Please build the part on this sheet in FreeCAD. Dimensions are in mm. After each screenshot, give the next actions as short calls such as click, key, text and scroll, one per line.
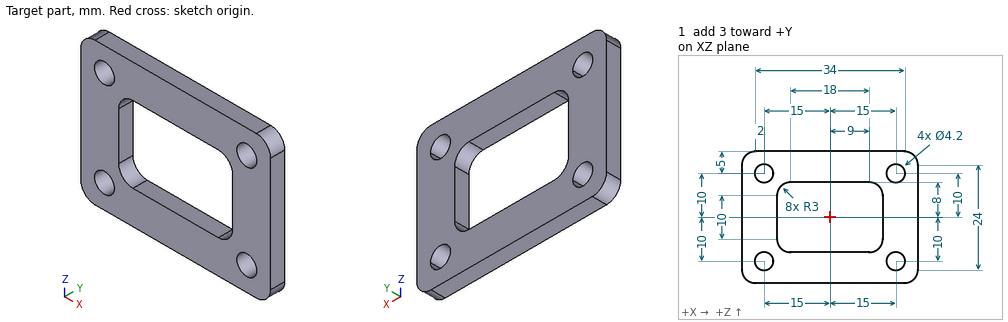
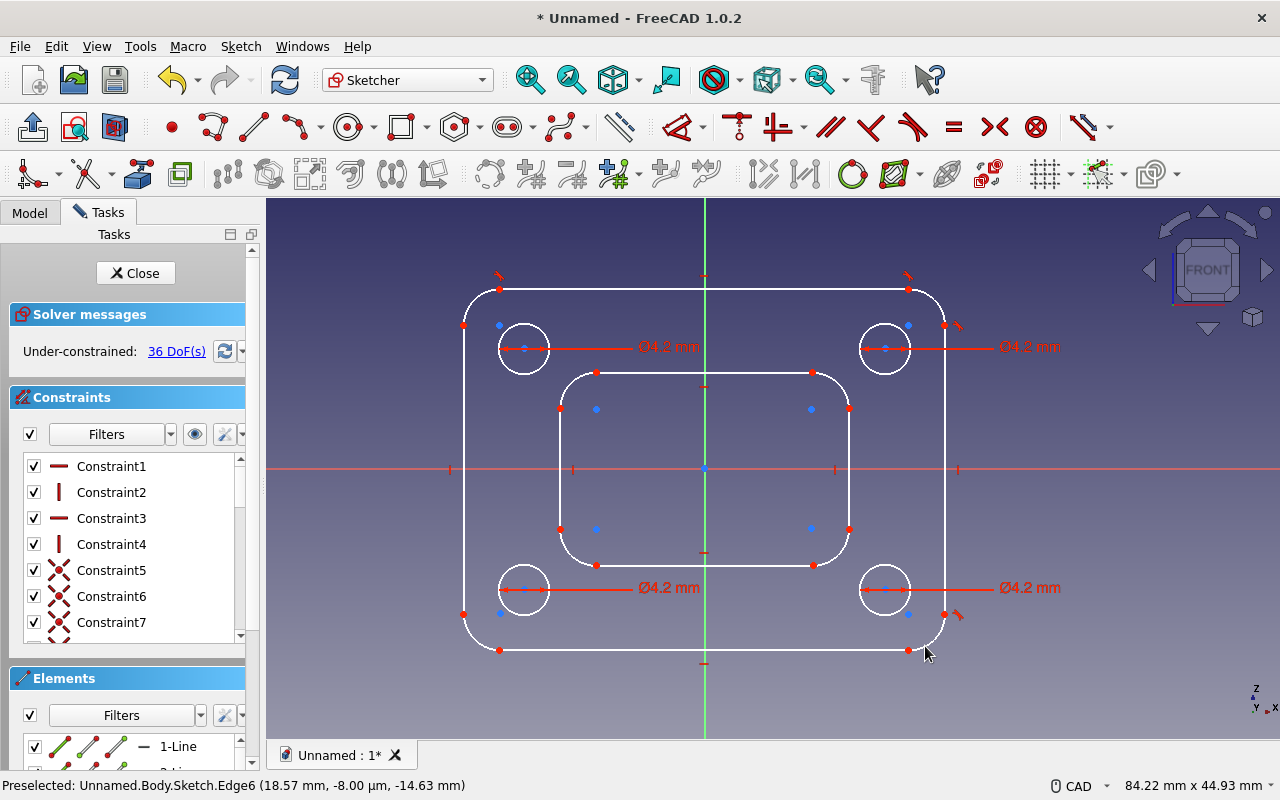
click(786, 650)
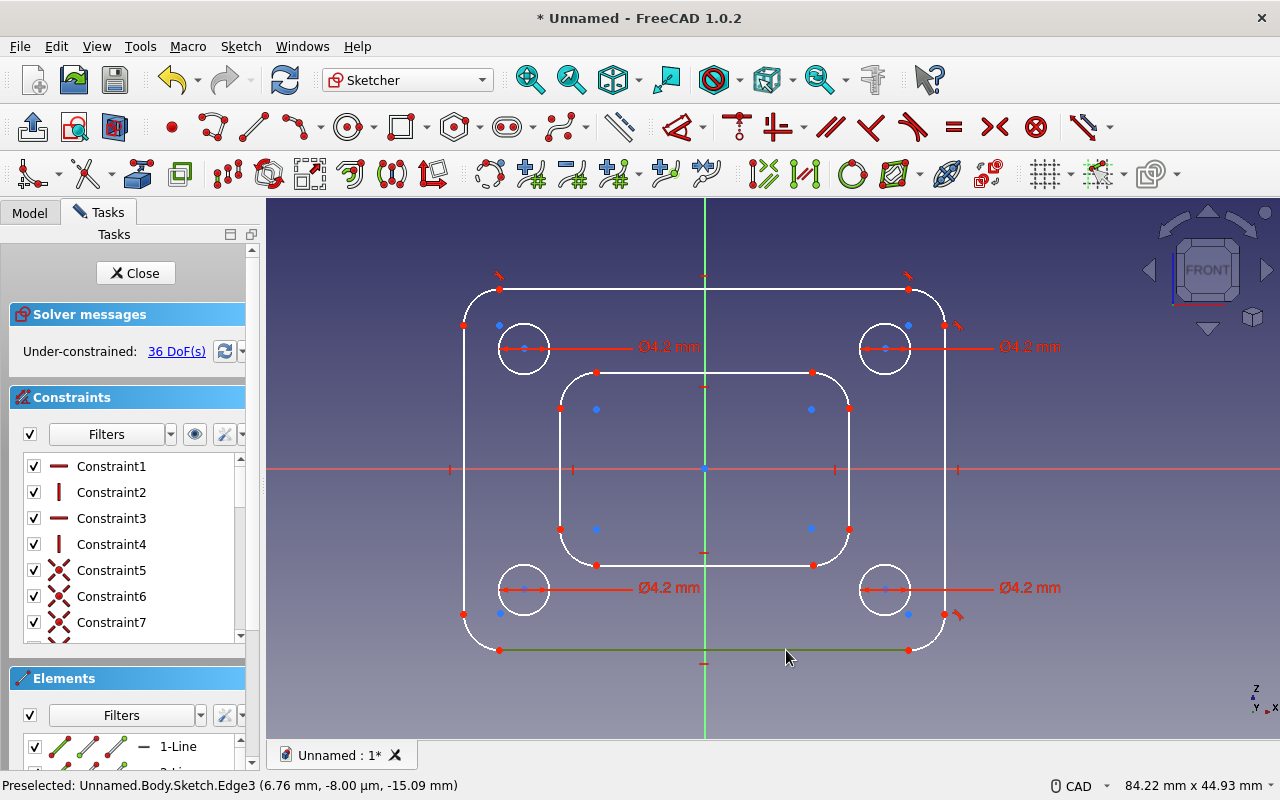
click(925, 646)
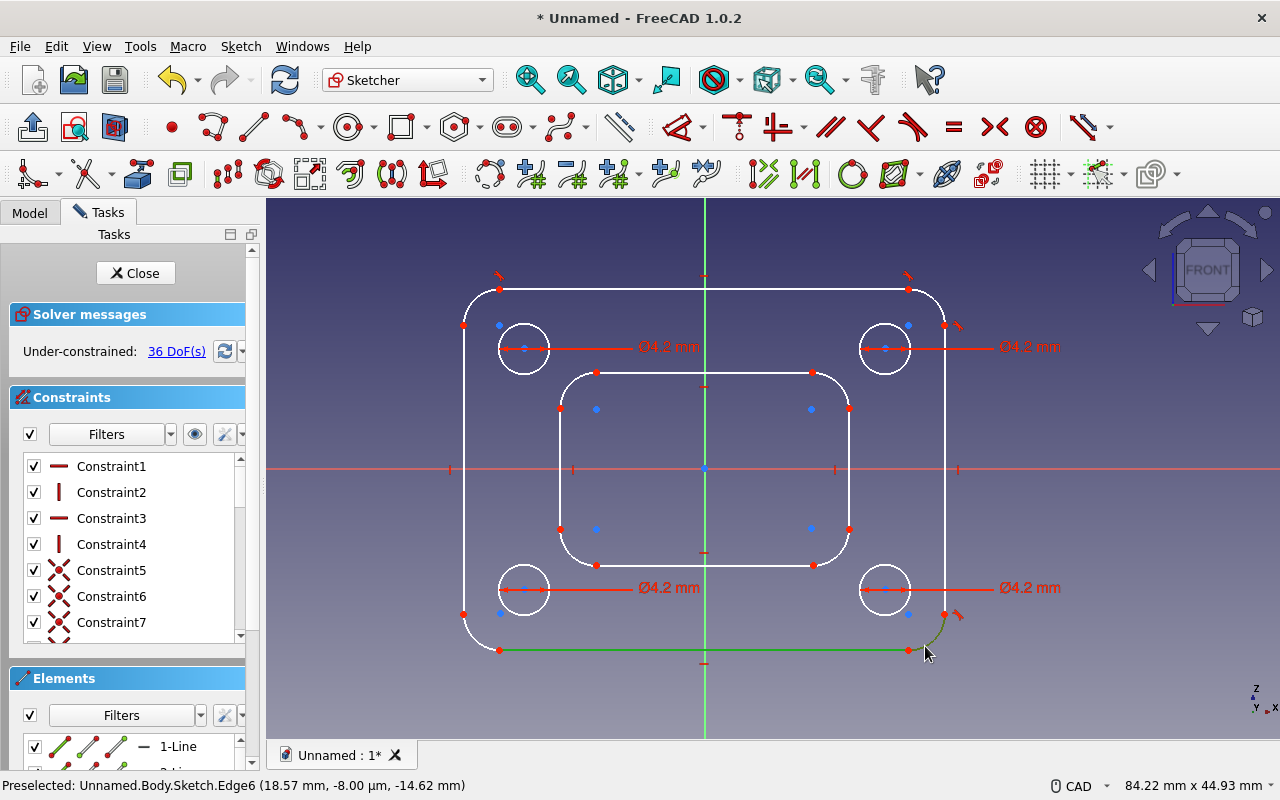
click(913, 128)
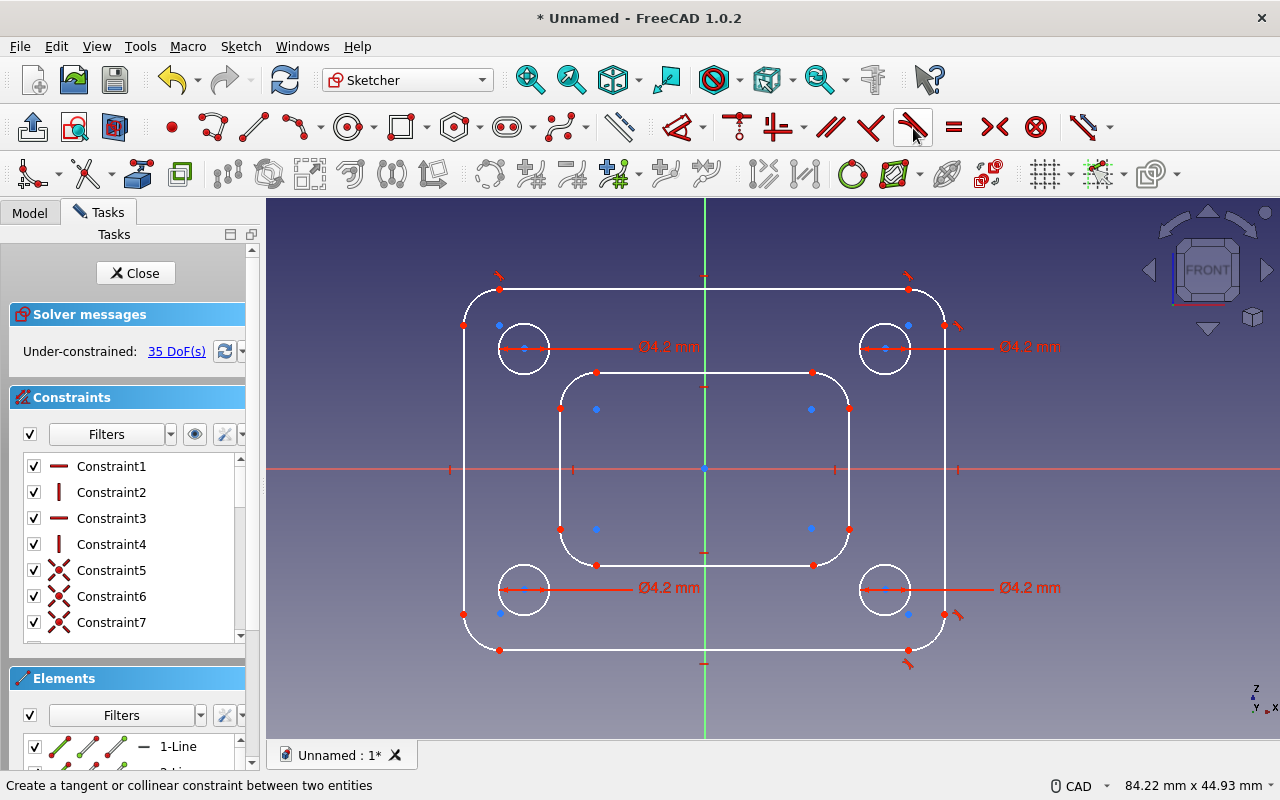
click(786, 650)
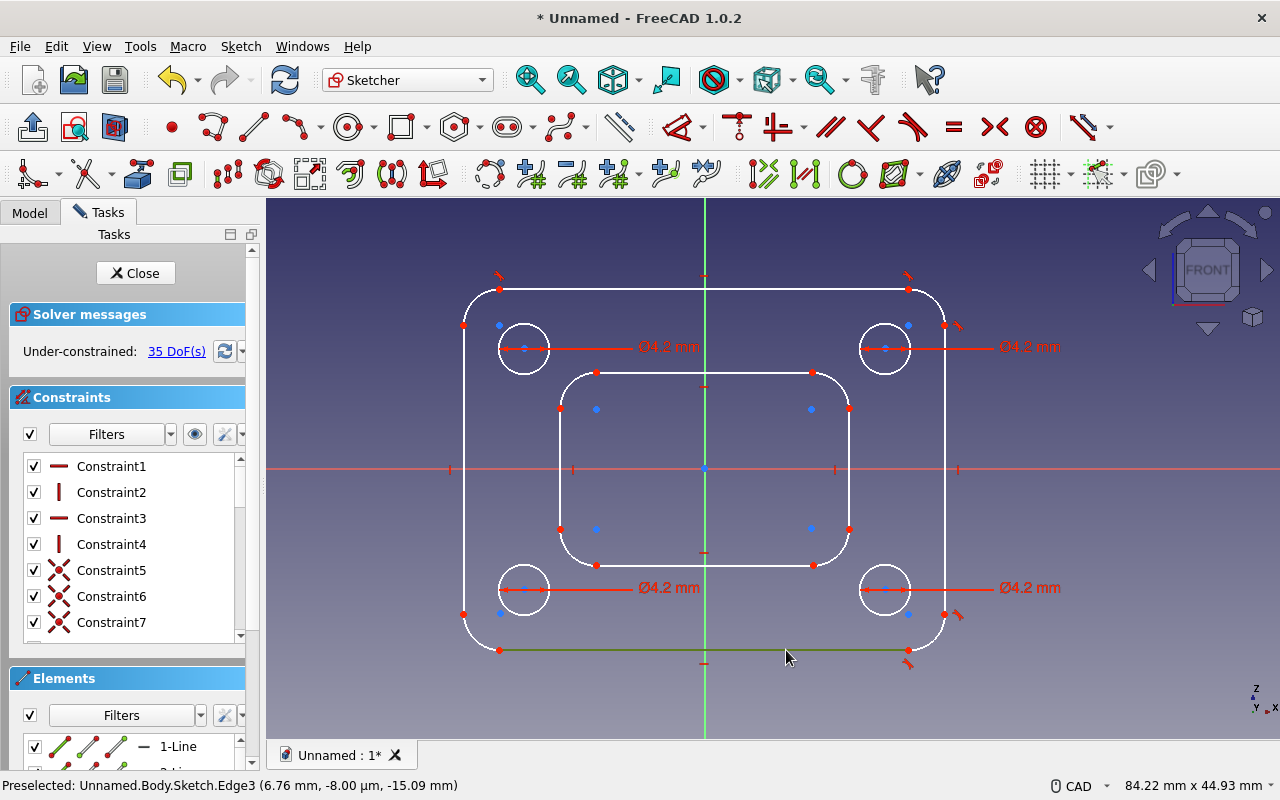
click(468, 631)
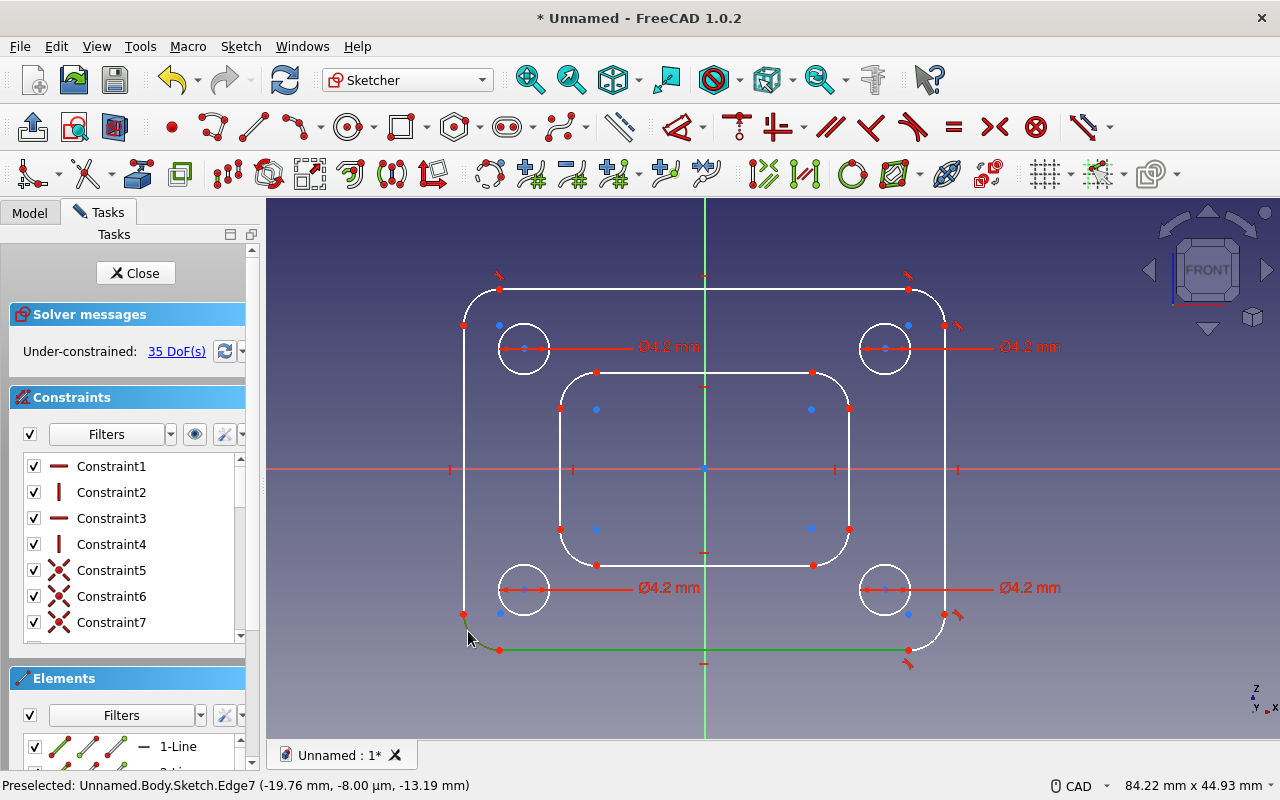
key(t)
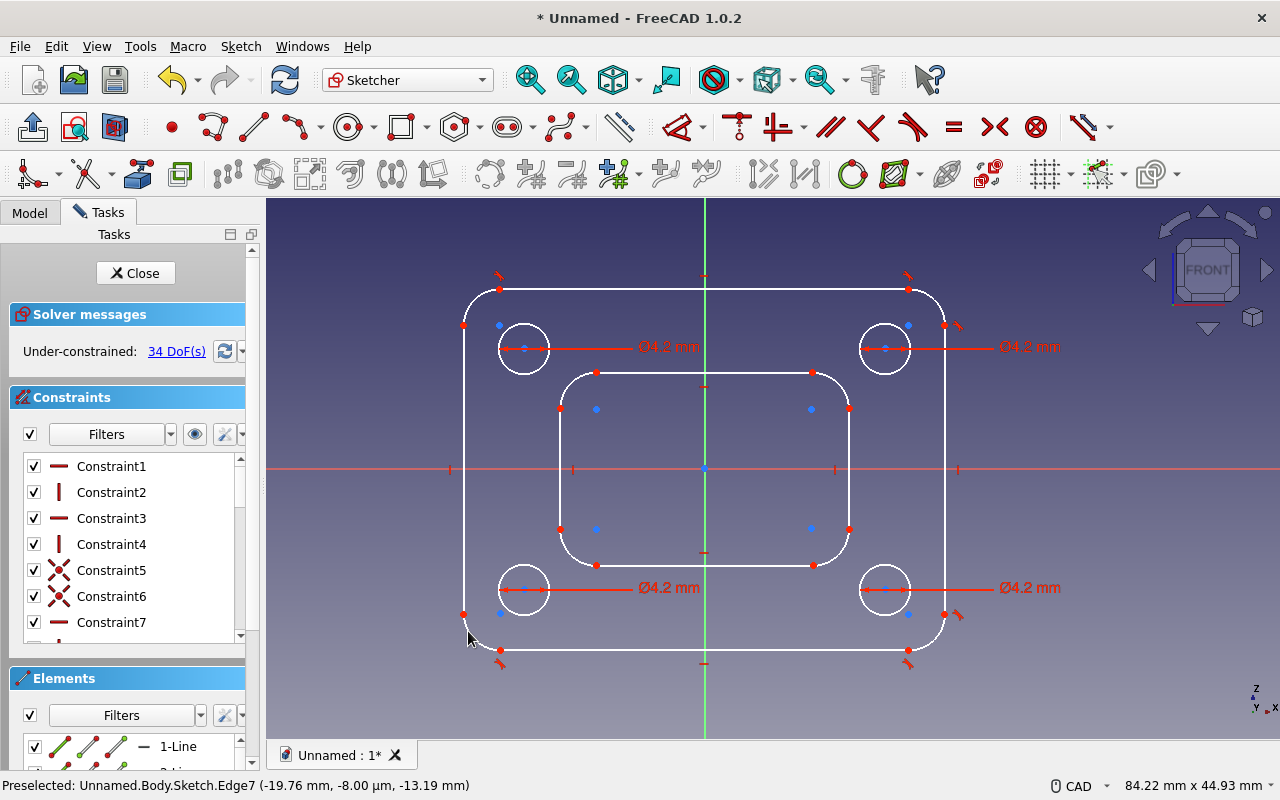
click(464, 528)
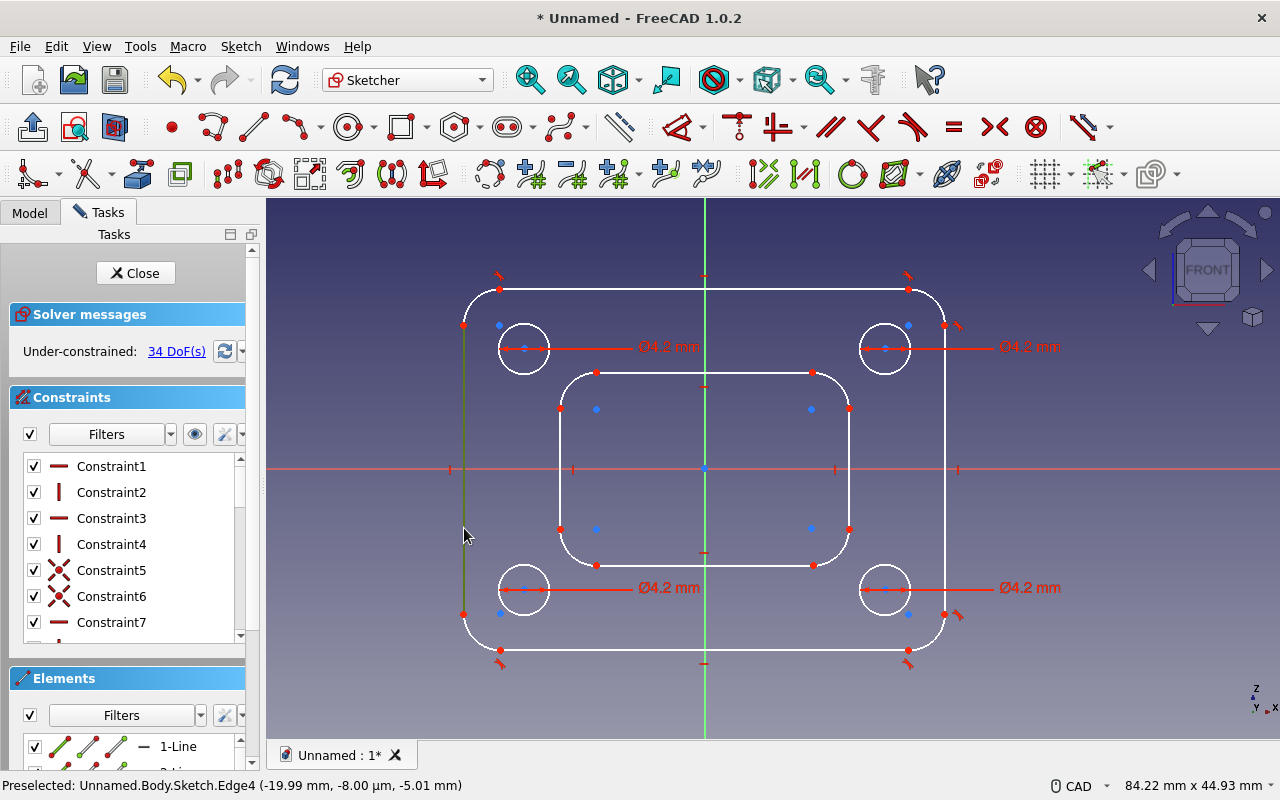
click(468, 631)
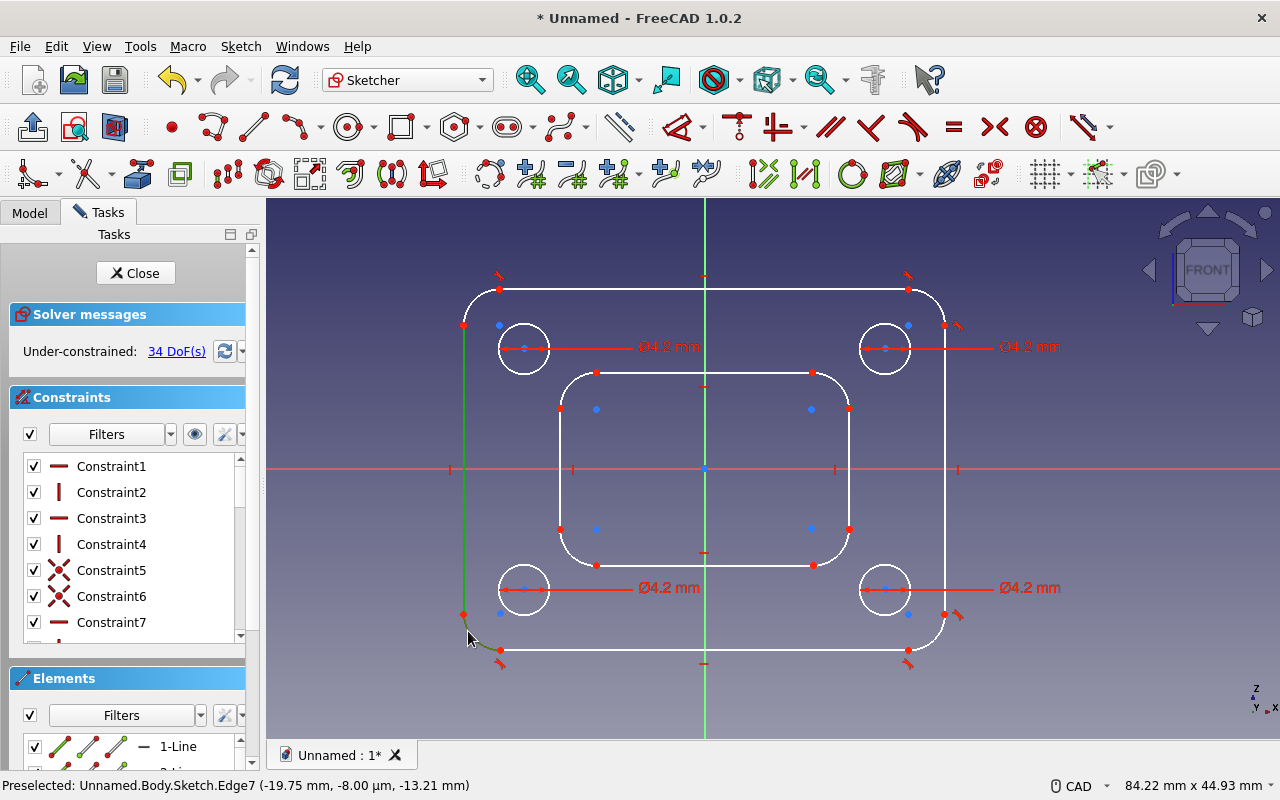
key(t)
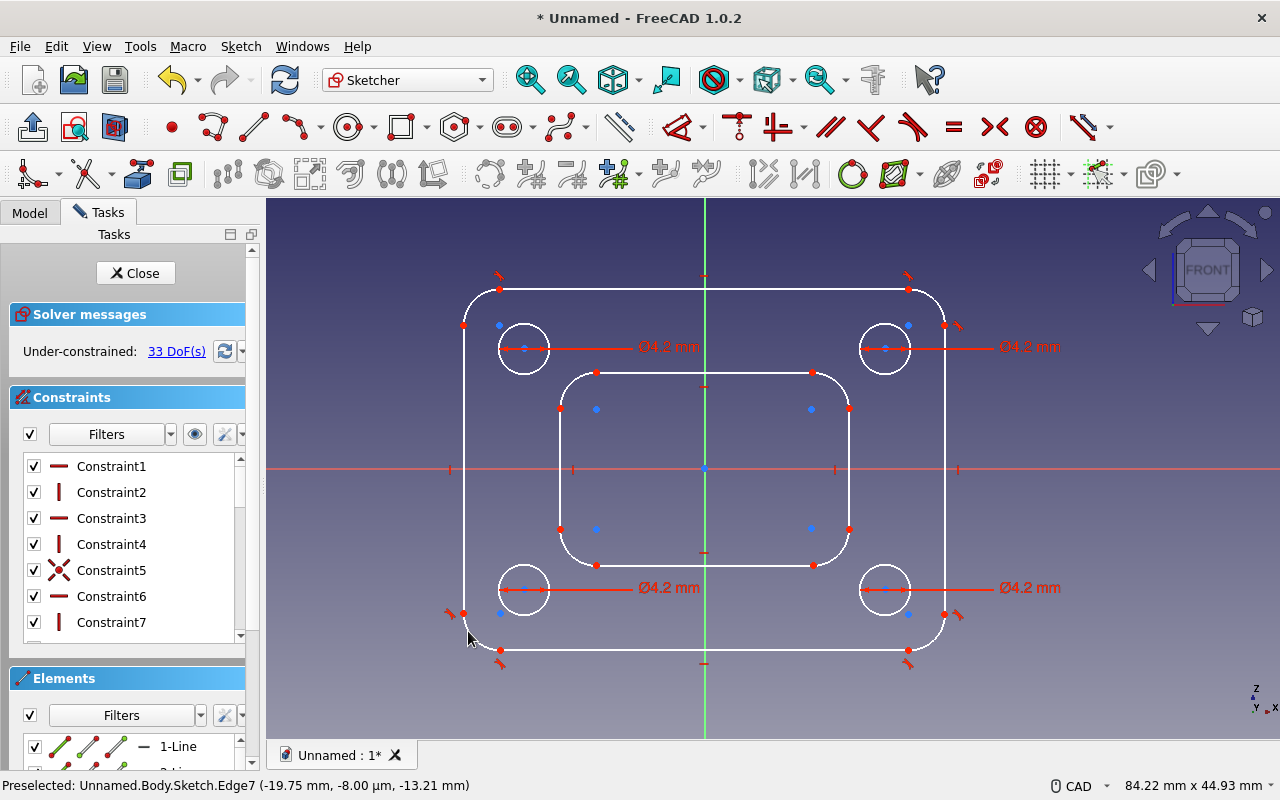
click(464, 527)